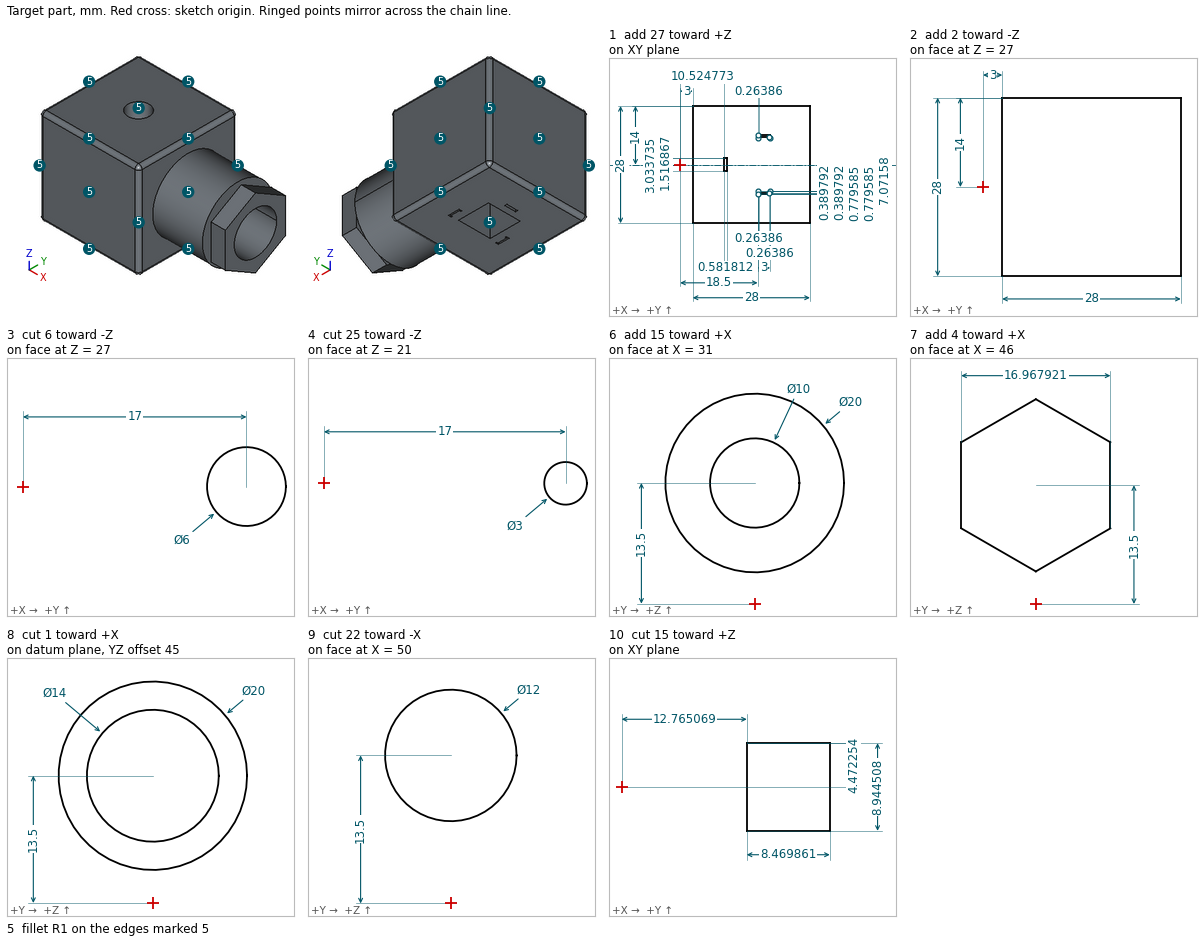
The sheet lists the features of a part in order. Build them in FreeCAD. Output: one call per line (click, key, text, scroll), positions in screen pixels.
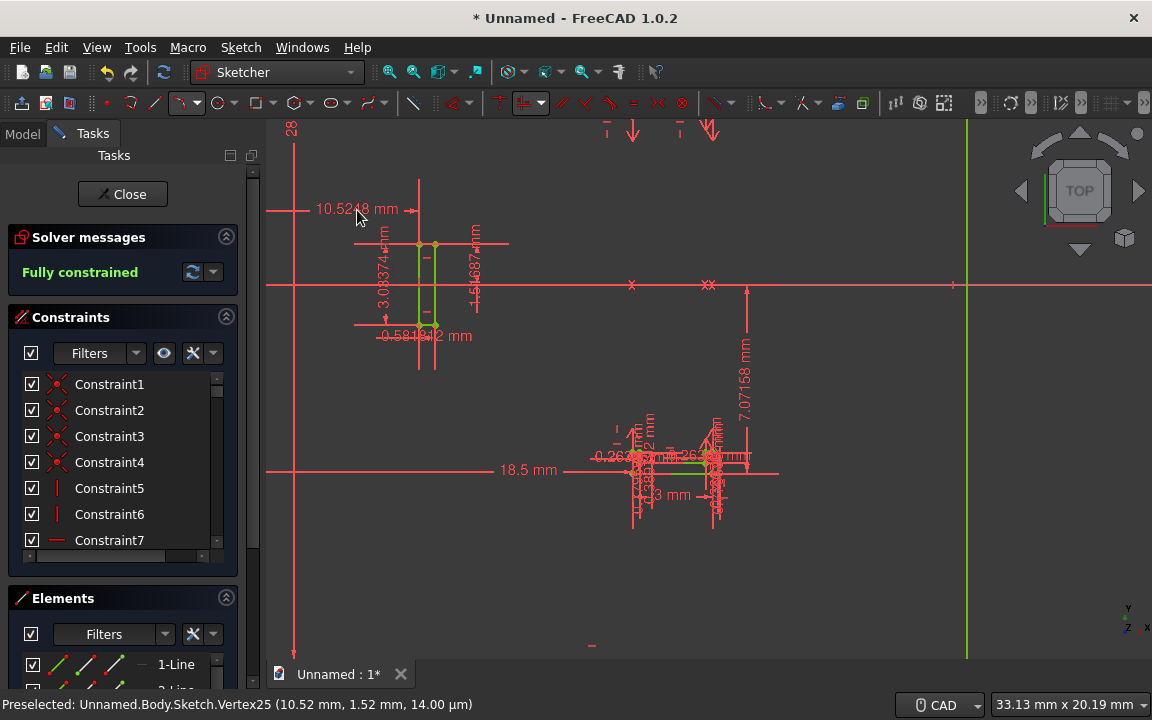
click(123, 194)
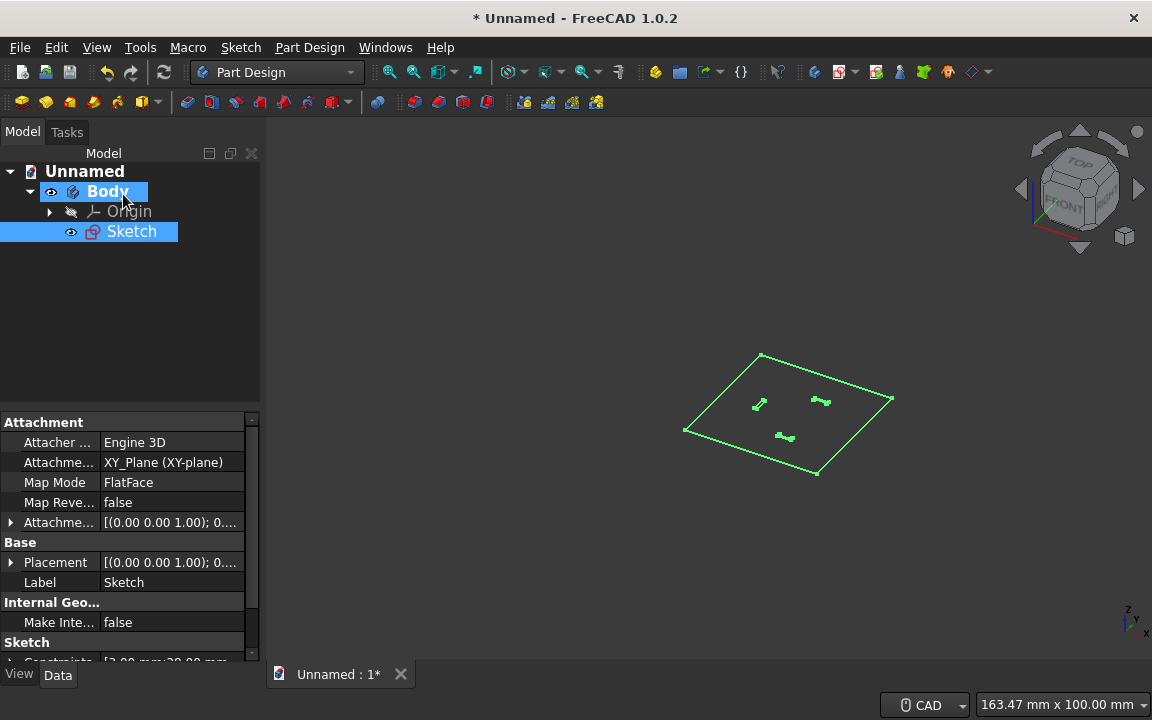
click(22, 102)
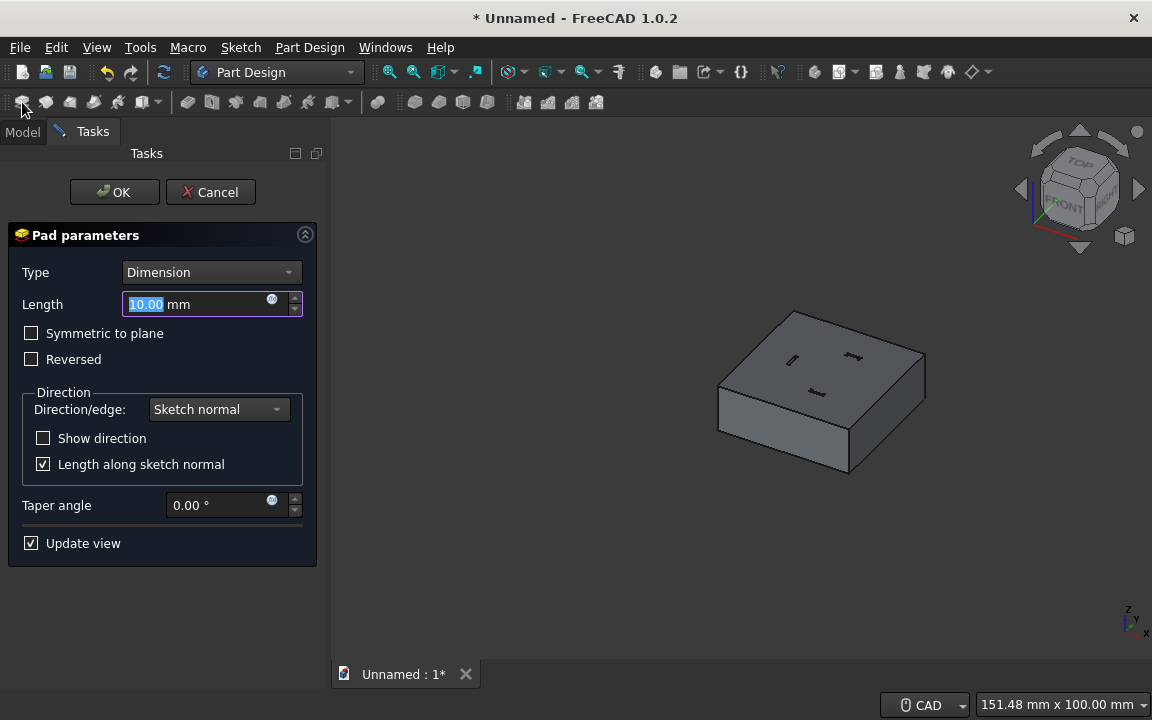
text(27)
key(Tab)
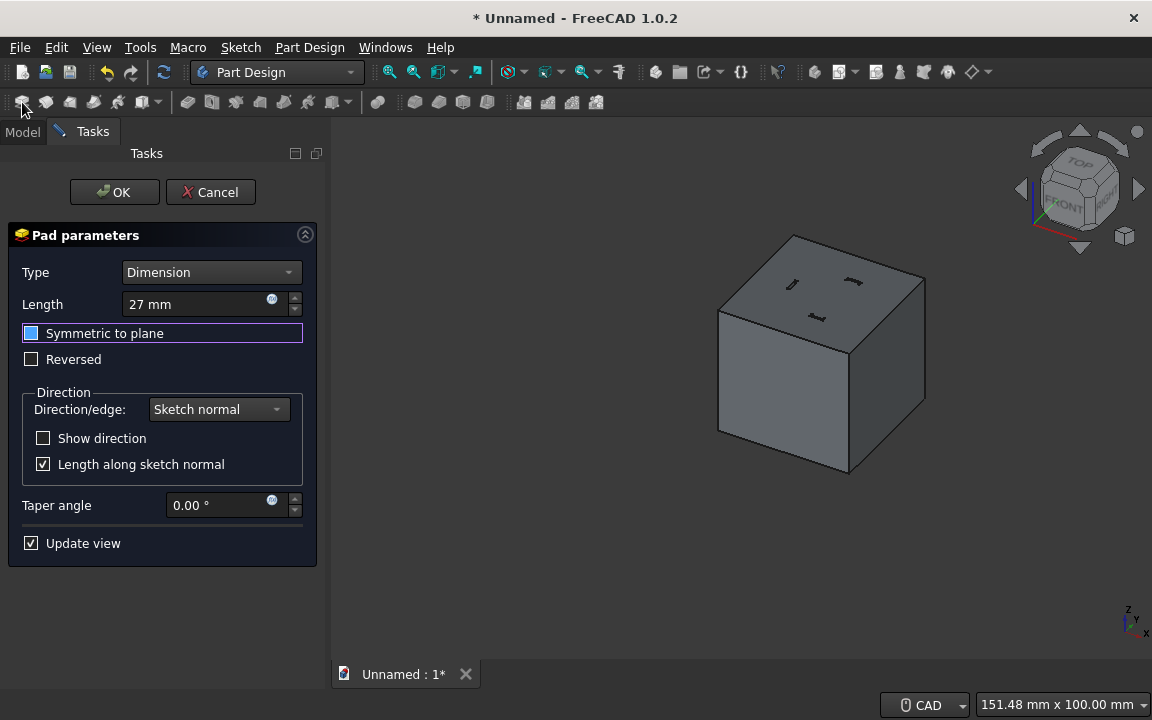
click(115, 192)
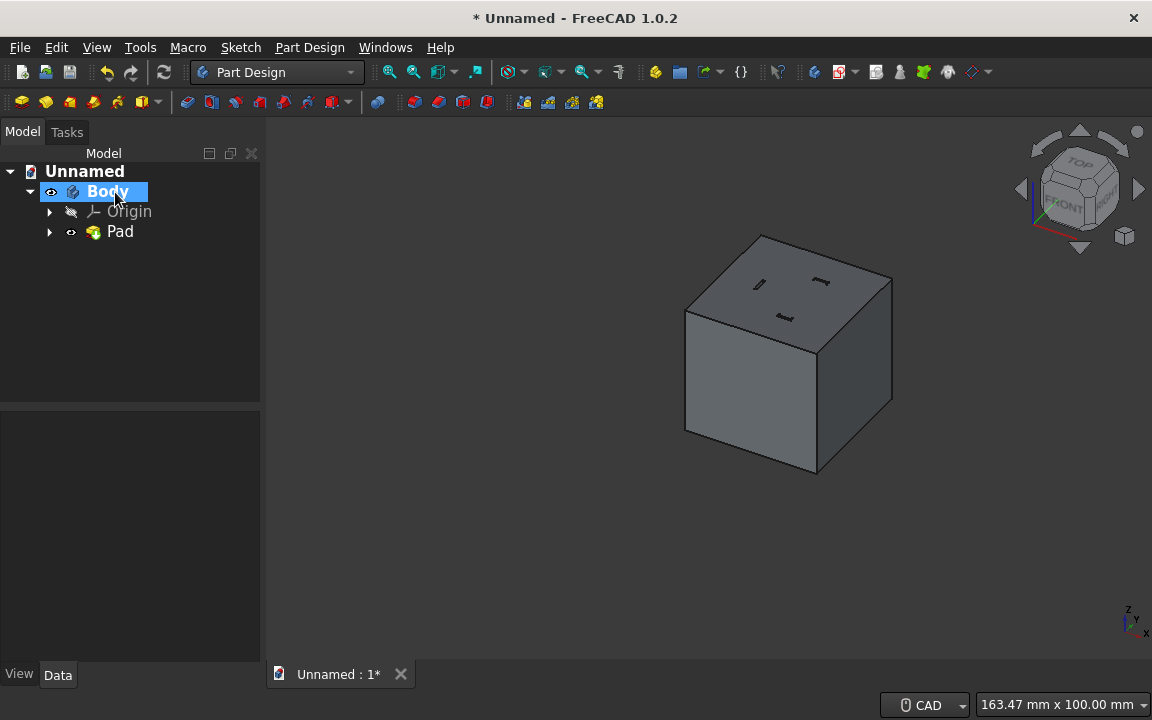
click(390, 72)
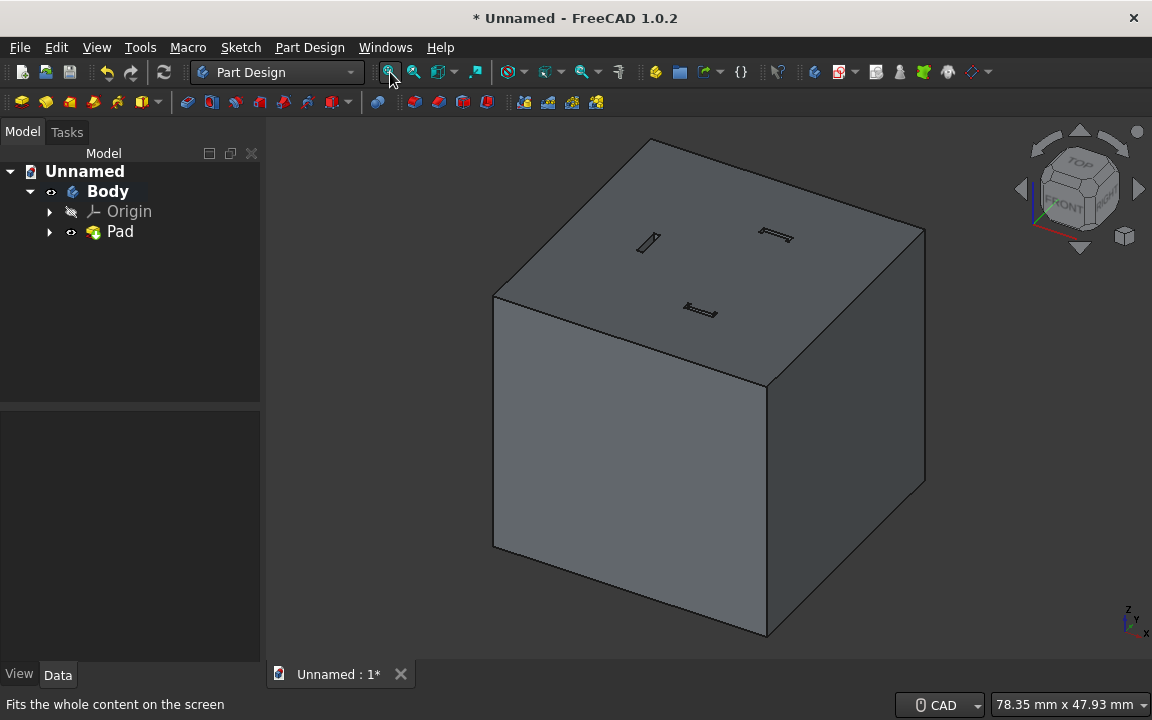
click(748, 275)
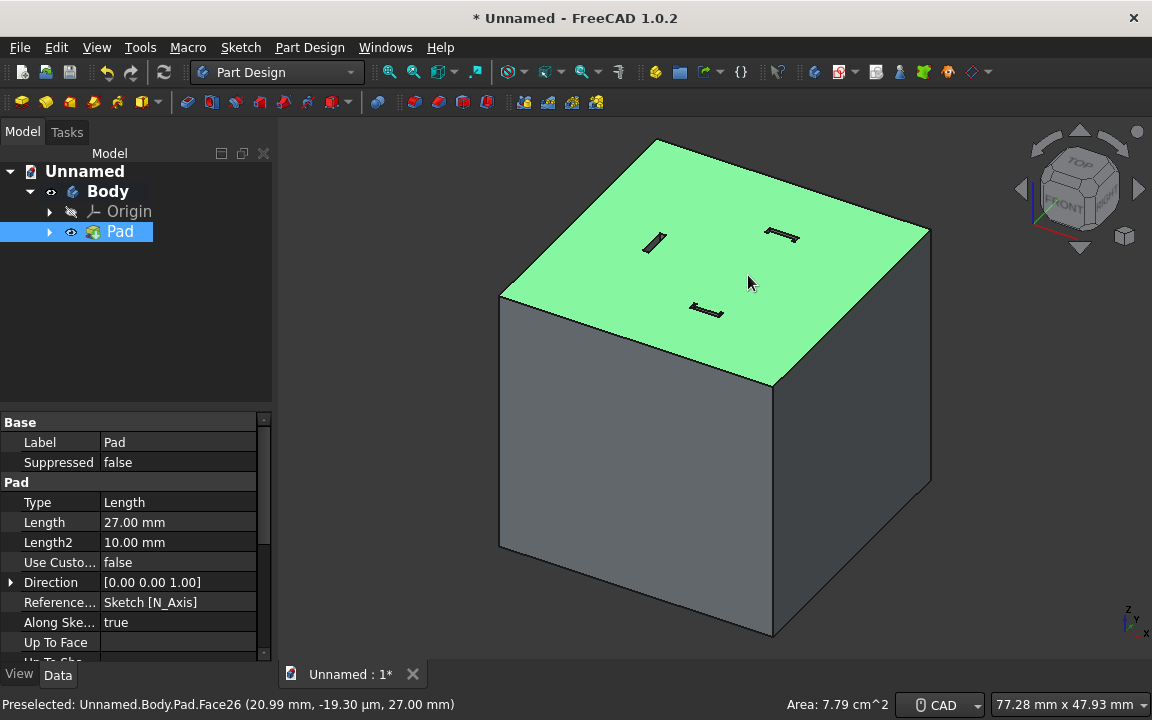
click(840, 72)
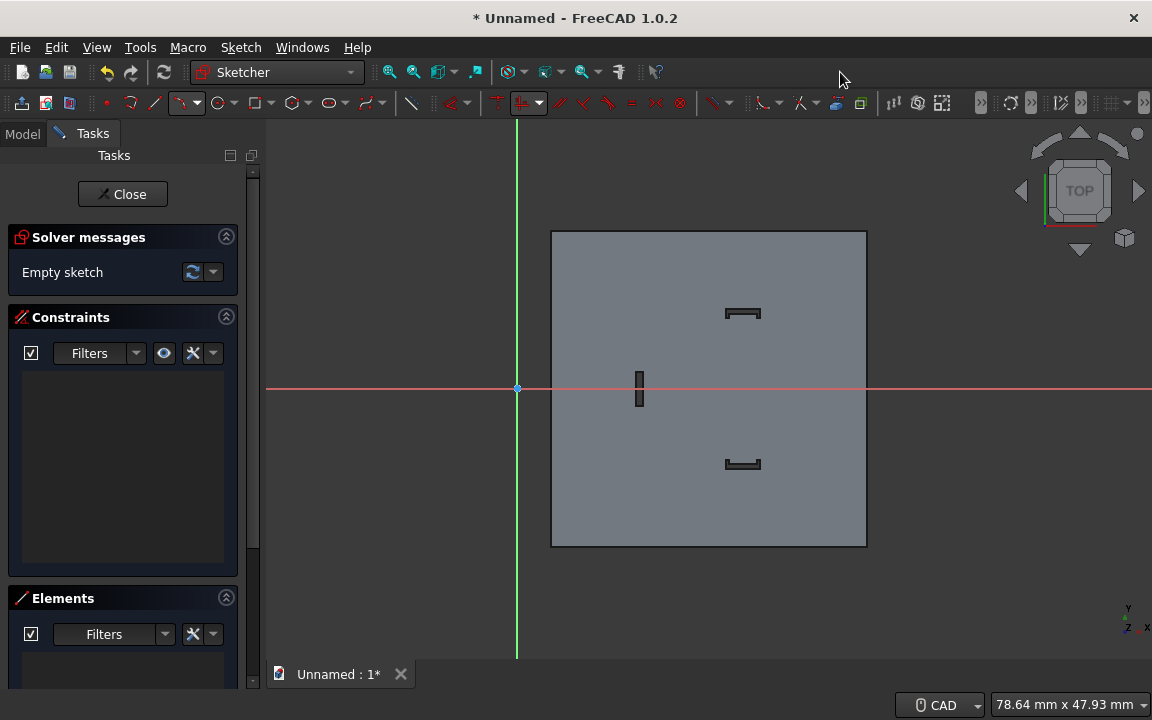
click(256, 104)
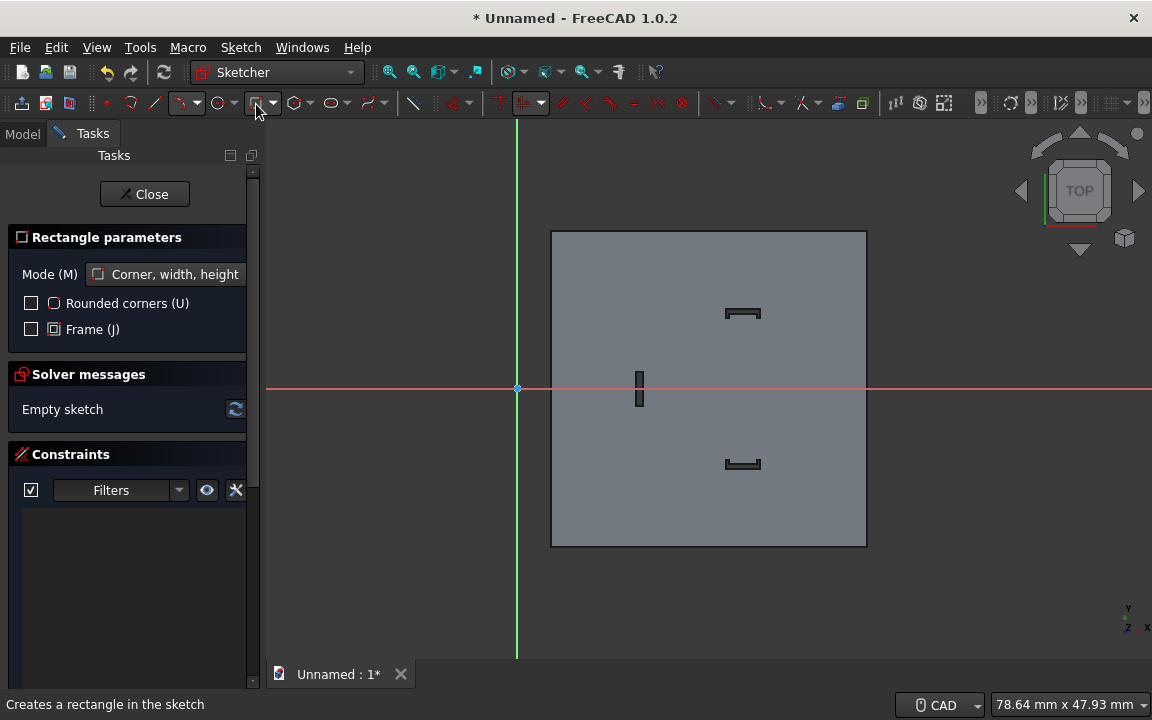
click(551, 231)
click(867, 547)
key(Escape)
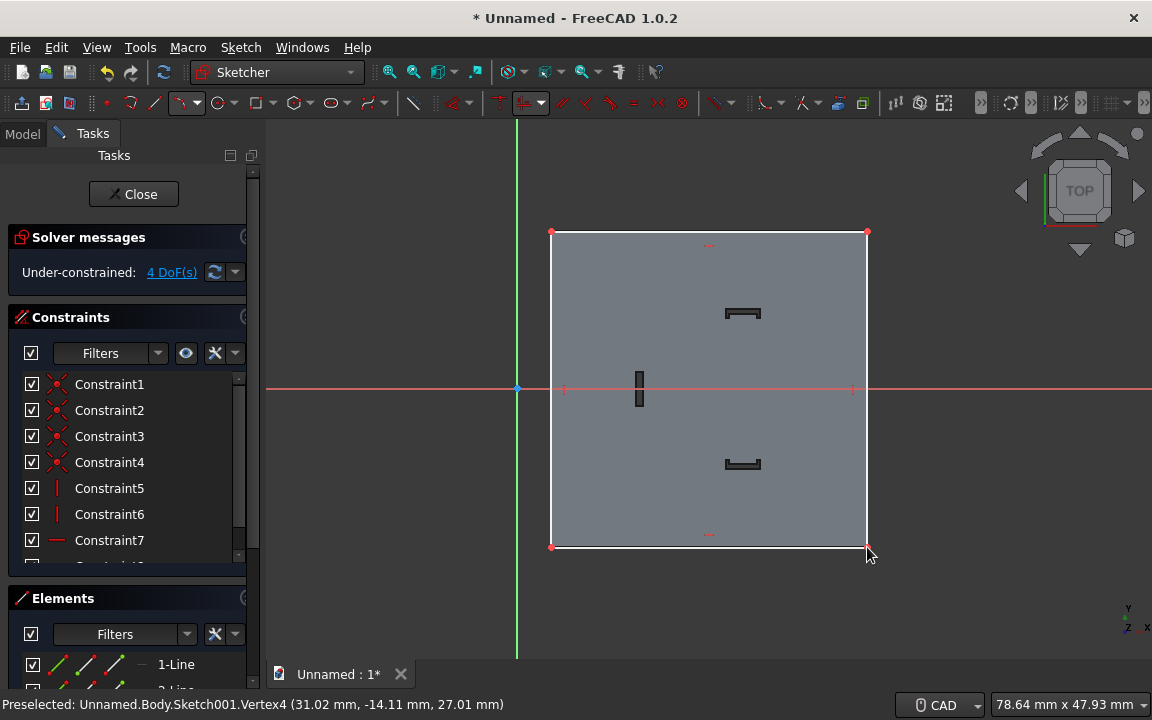
click(452, 104)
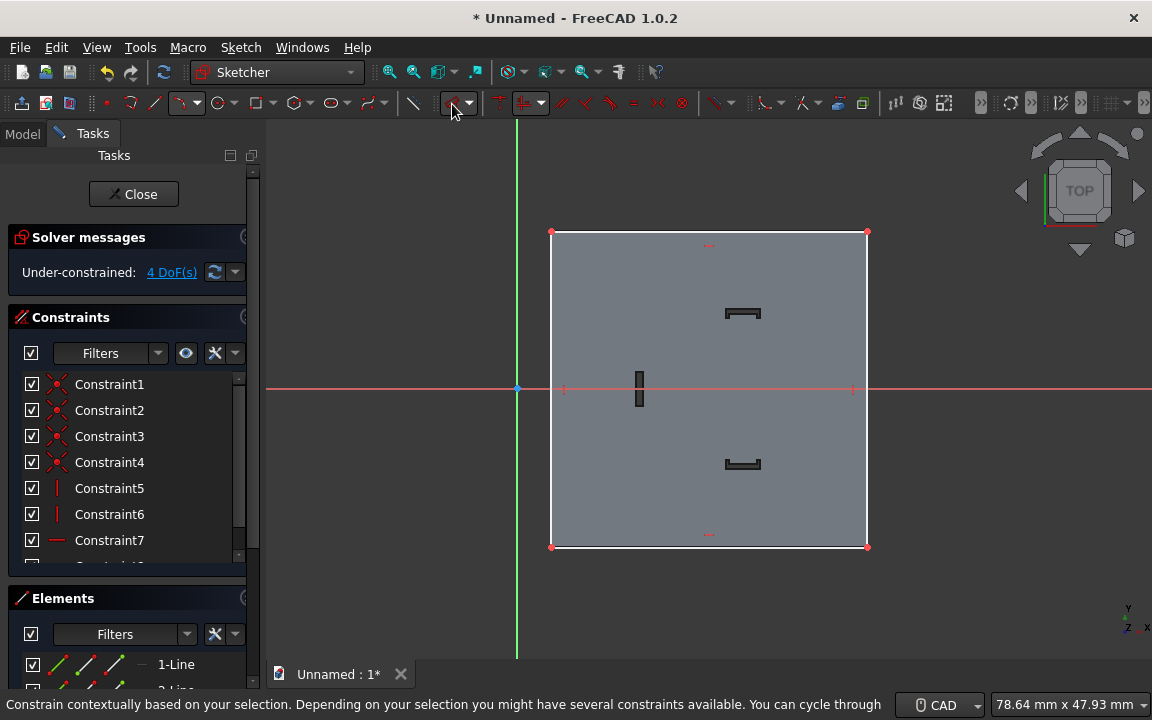
click(551, 327)
click(585, 317)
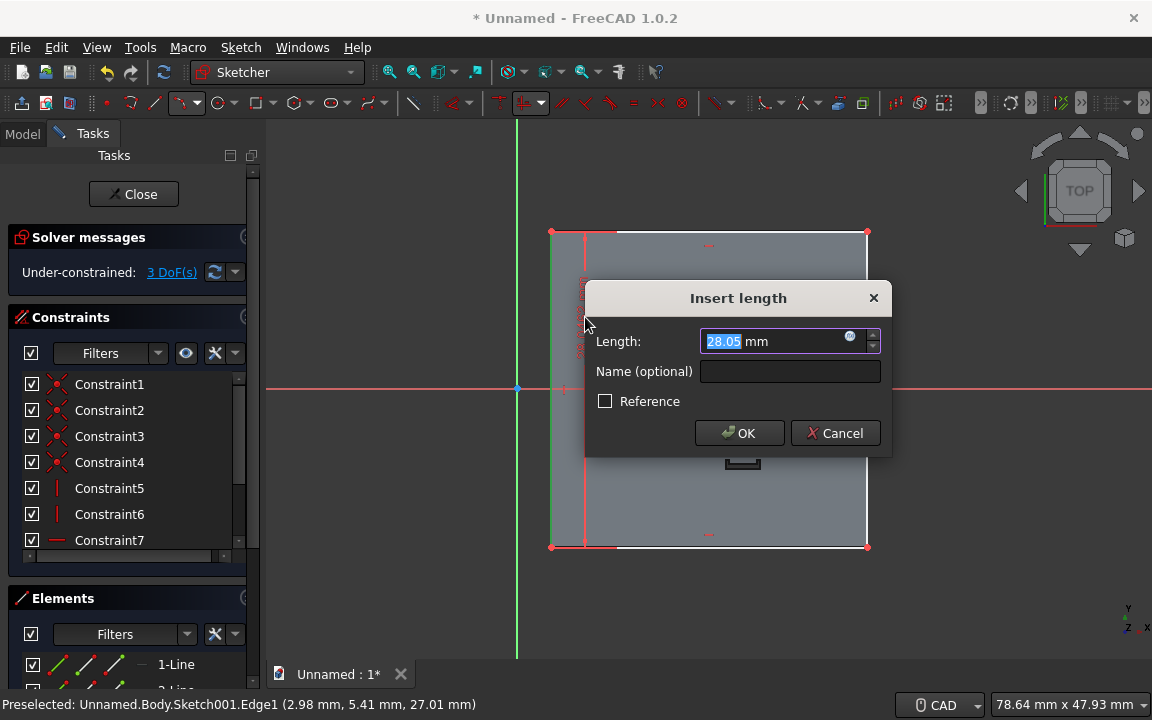
text(28)
key(Return)